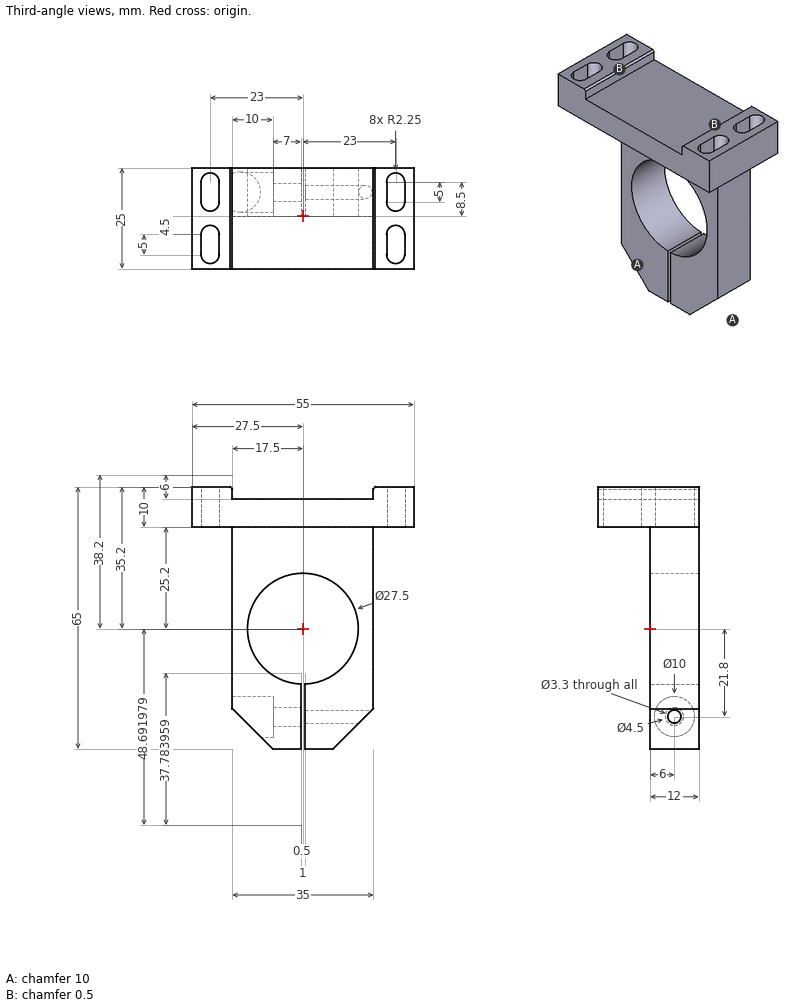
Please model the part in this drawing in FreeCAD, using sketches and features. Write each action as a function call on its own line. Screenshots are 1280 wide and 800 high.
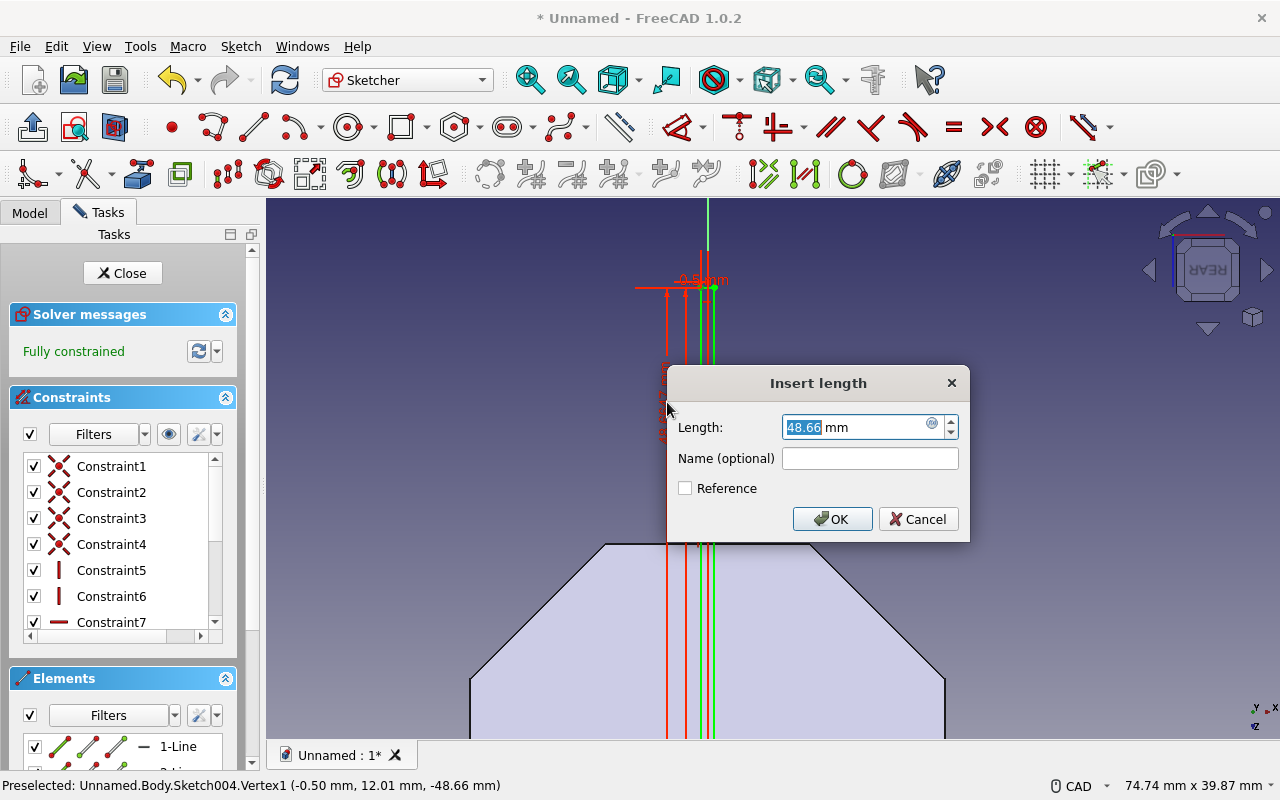
text(48.691979)
key(Return)
key(Escape)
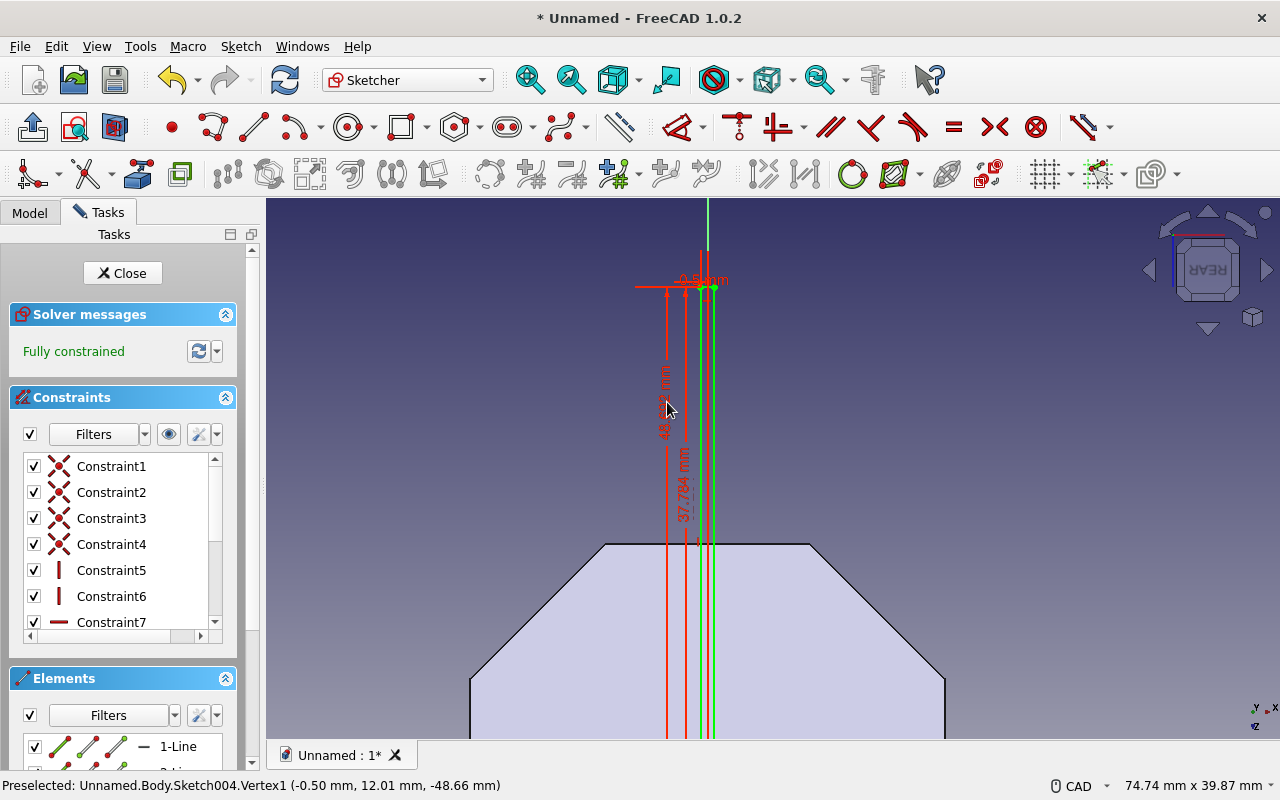
click(123, 273)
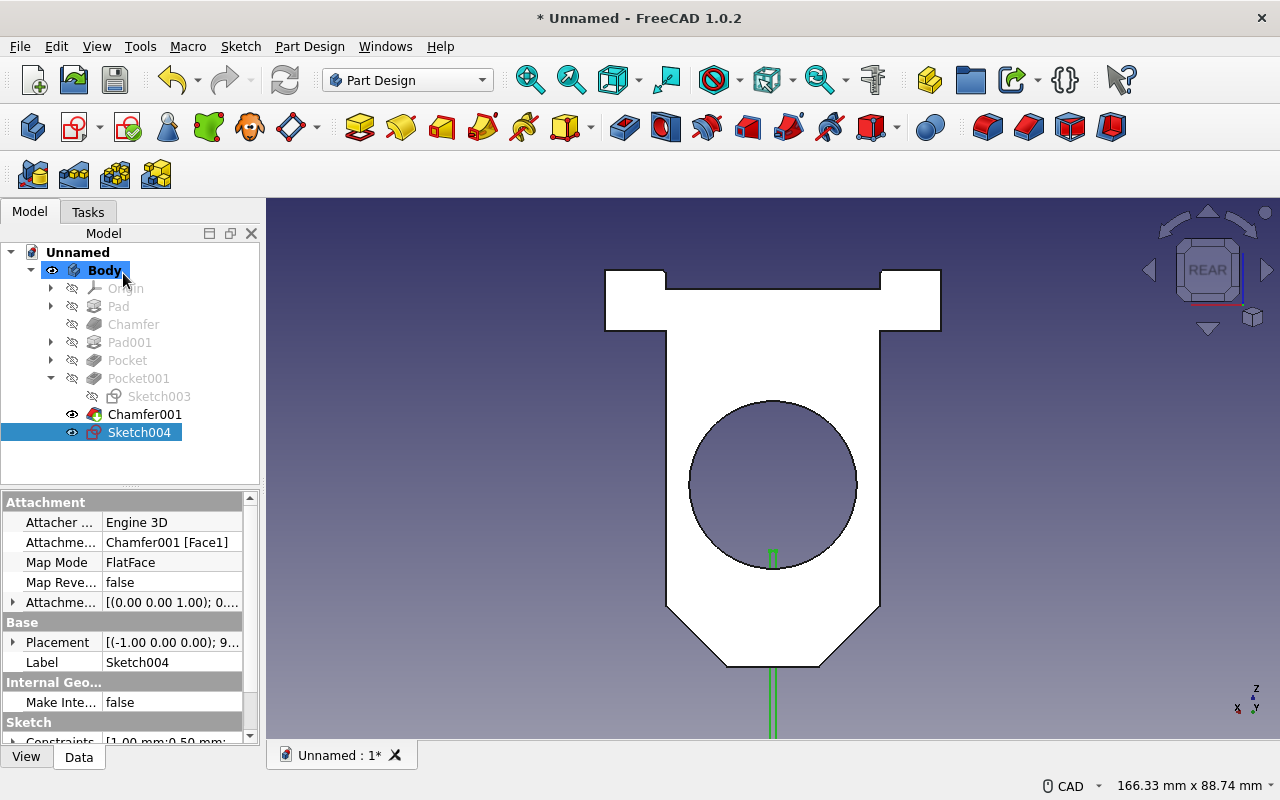
click(625, 128)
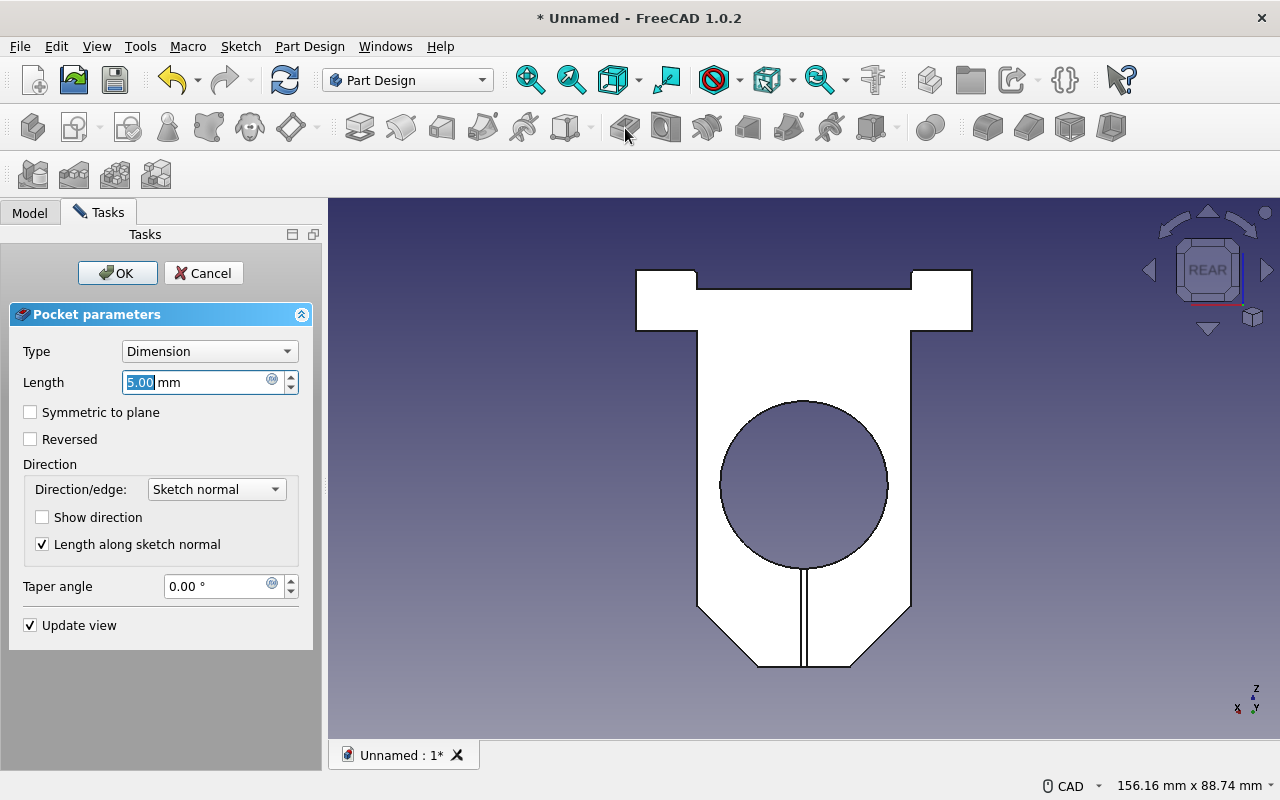
click(210, 352)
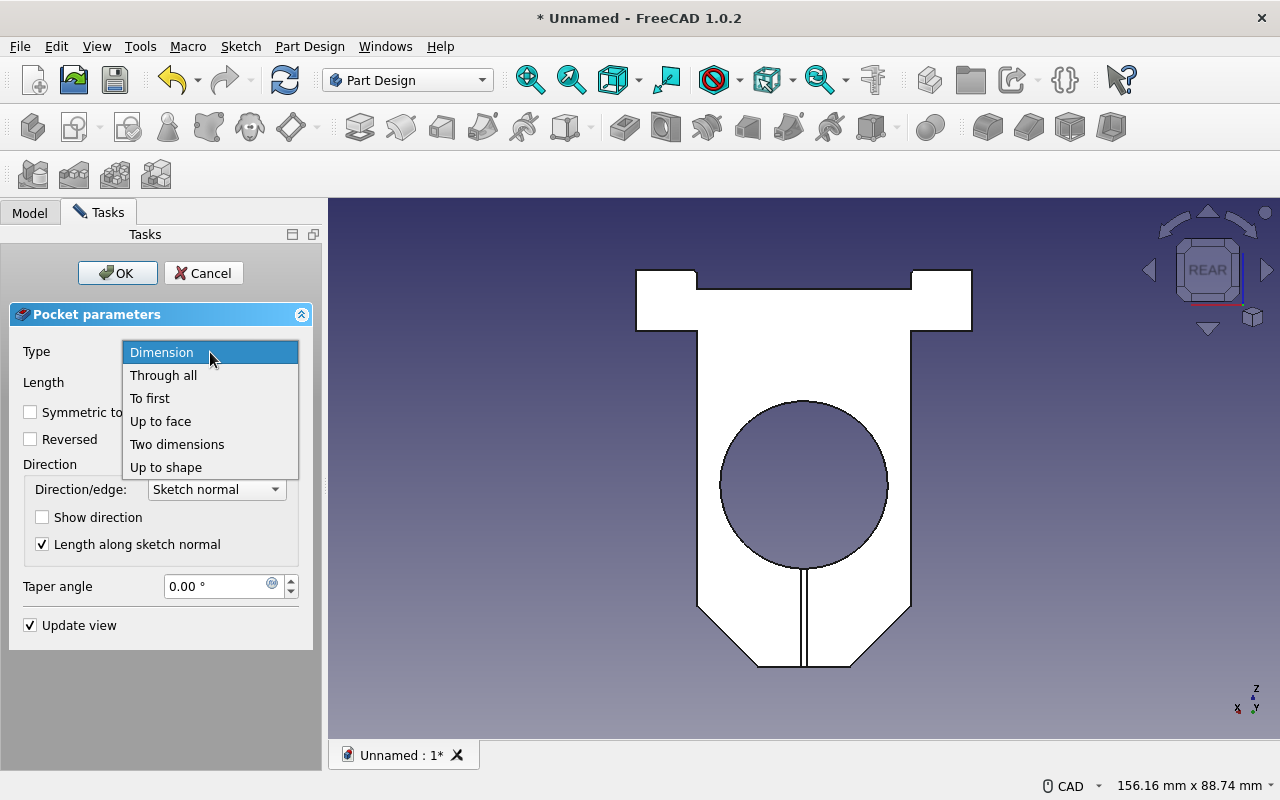
click(208, 376)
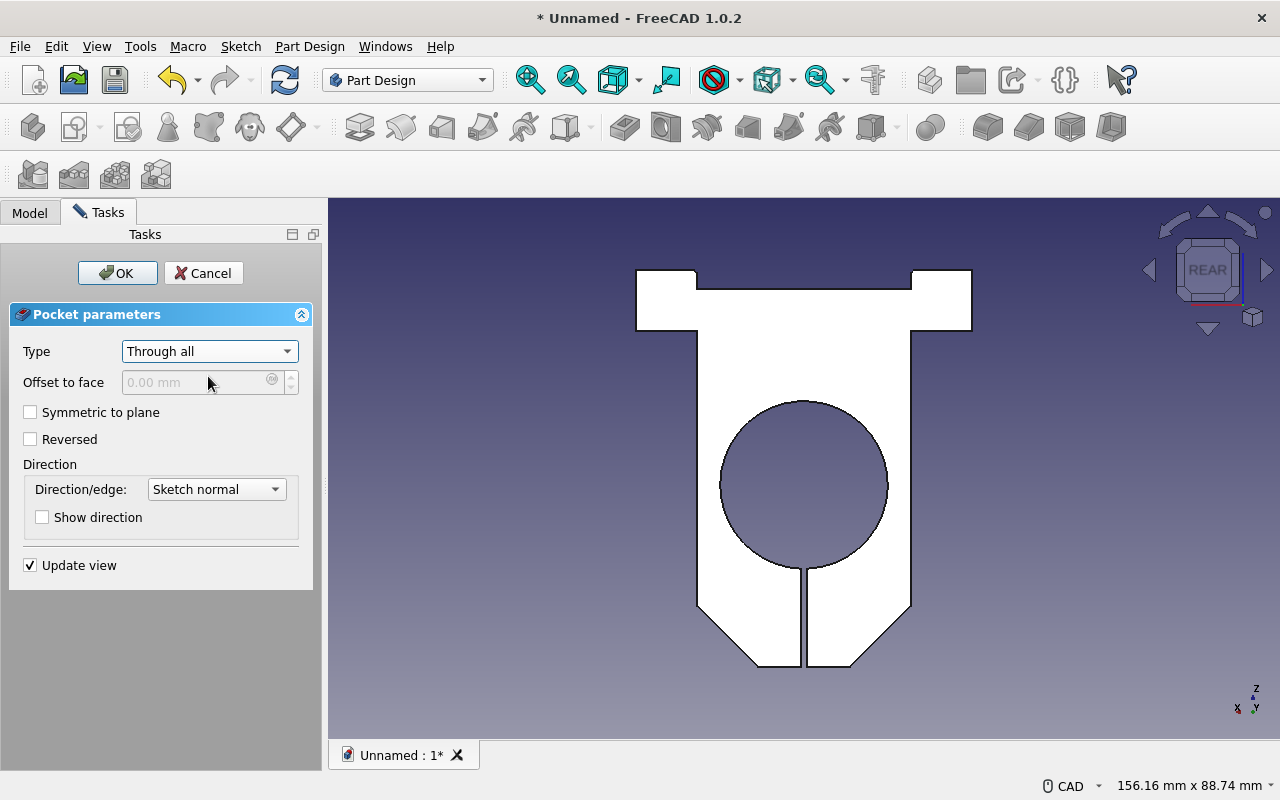
click(118, 273)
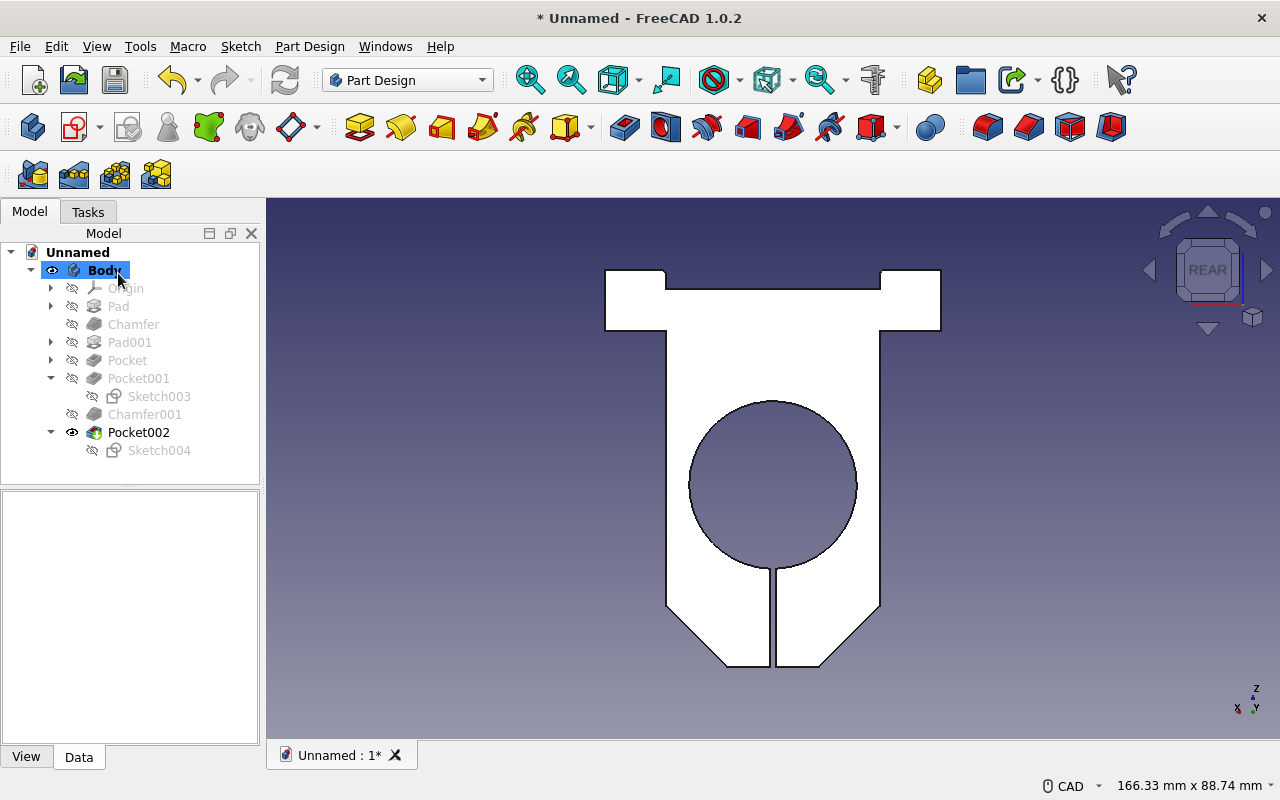
key(6)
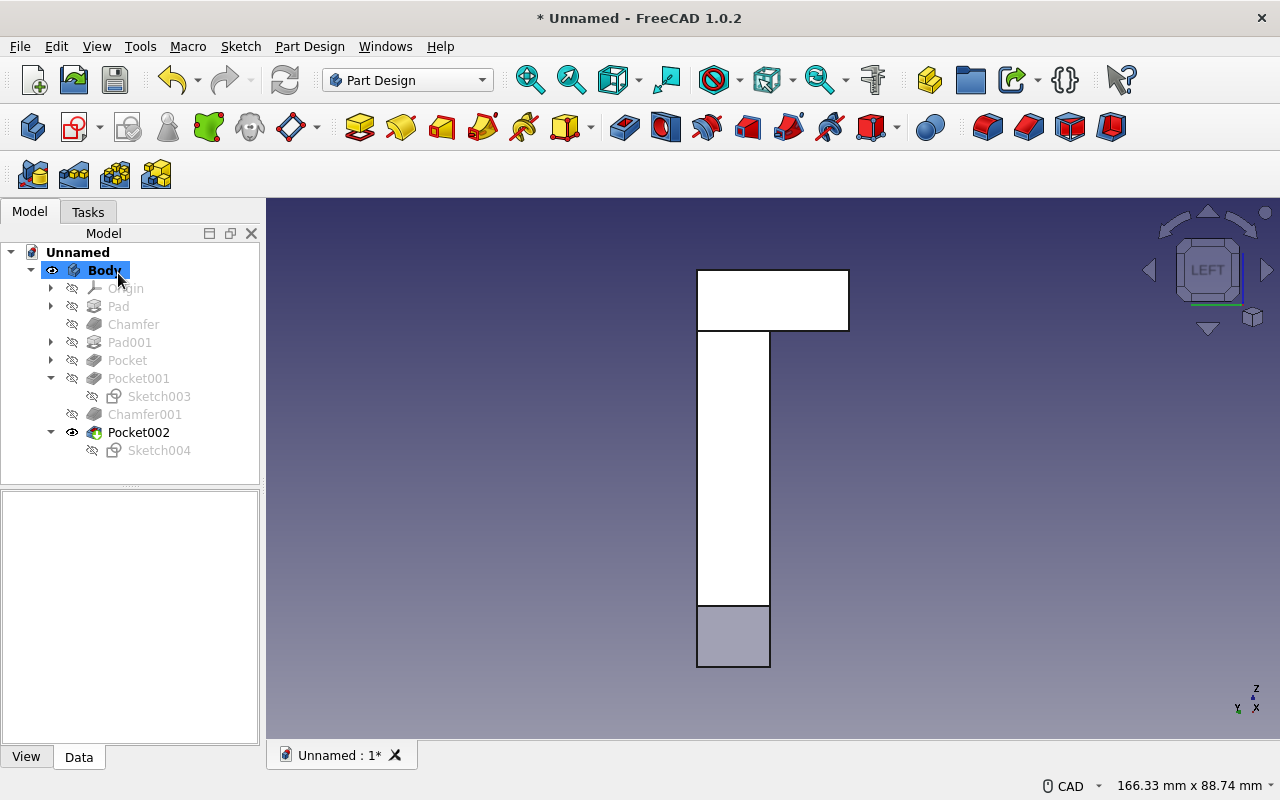
click(733, 389)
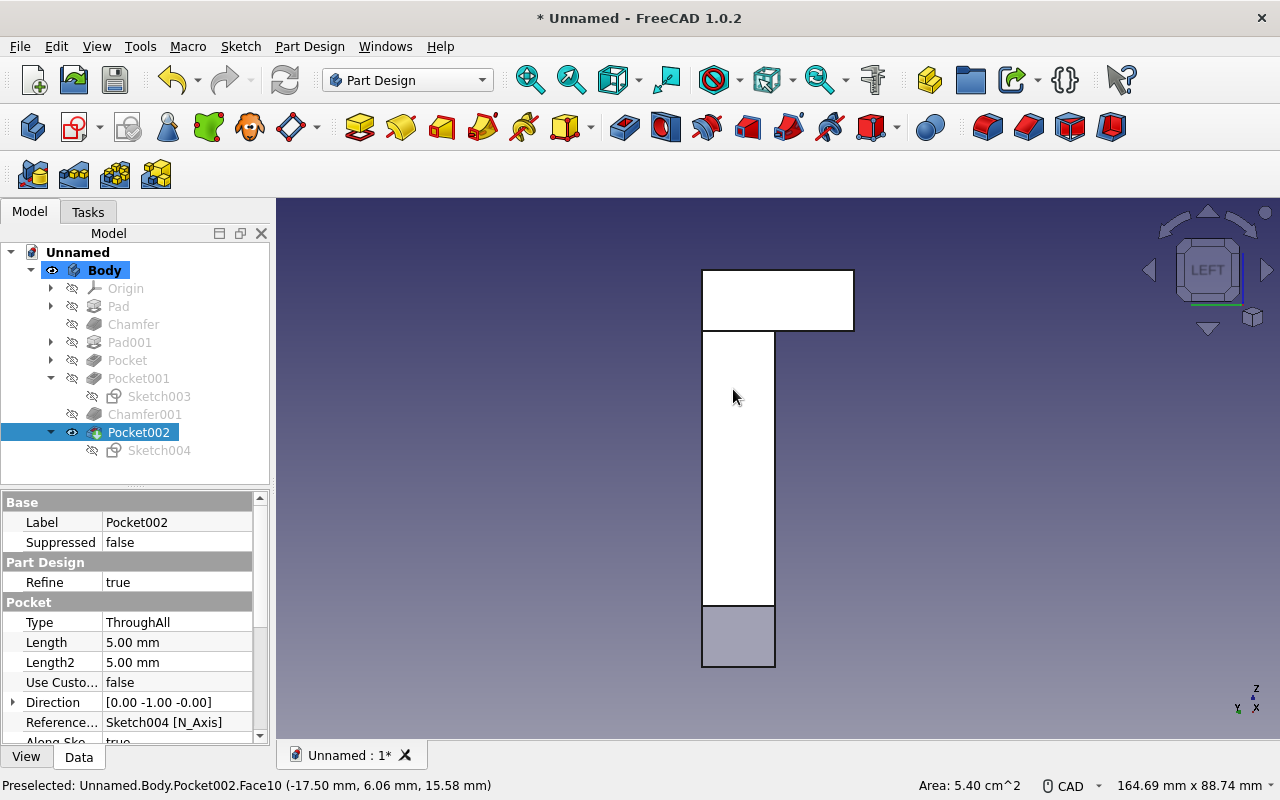
click(74, 128)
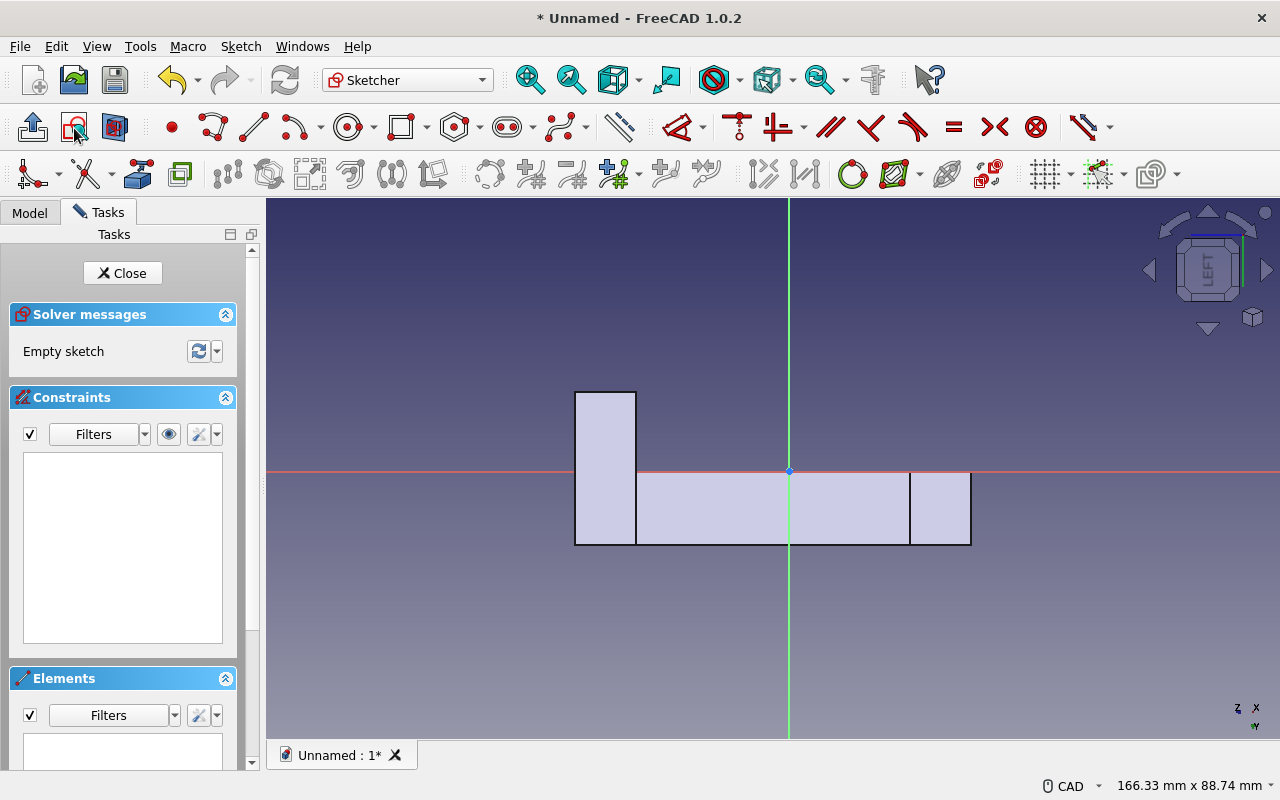
scroll(966, 516, up, 9)